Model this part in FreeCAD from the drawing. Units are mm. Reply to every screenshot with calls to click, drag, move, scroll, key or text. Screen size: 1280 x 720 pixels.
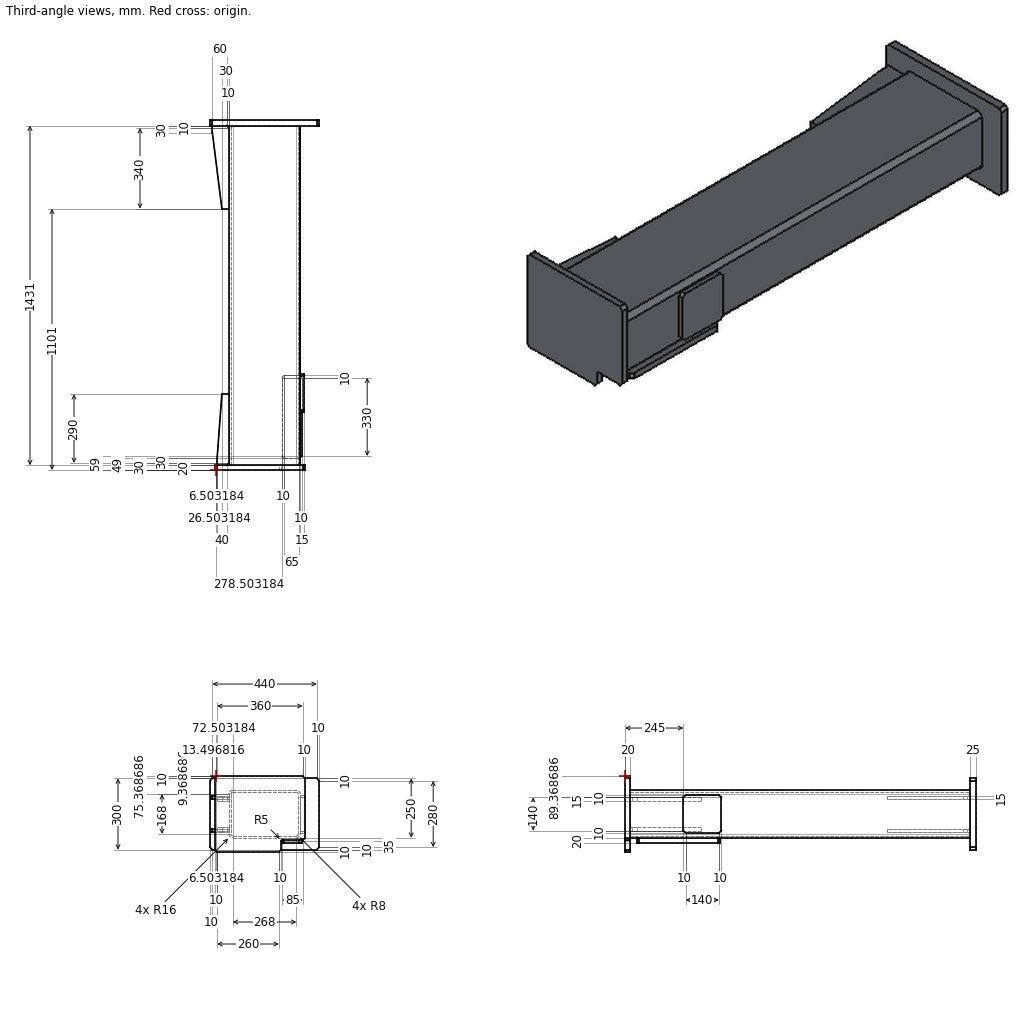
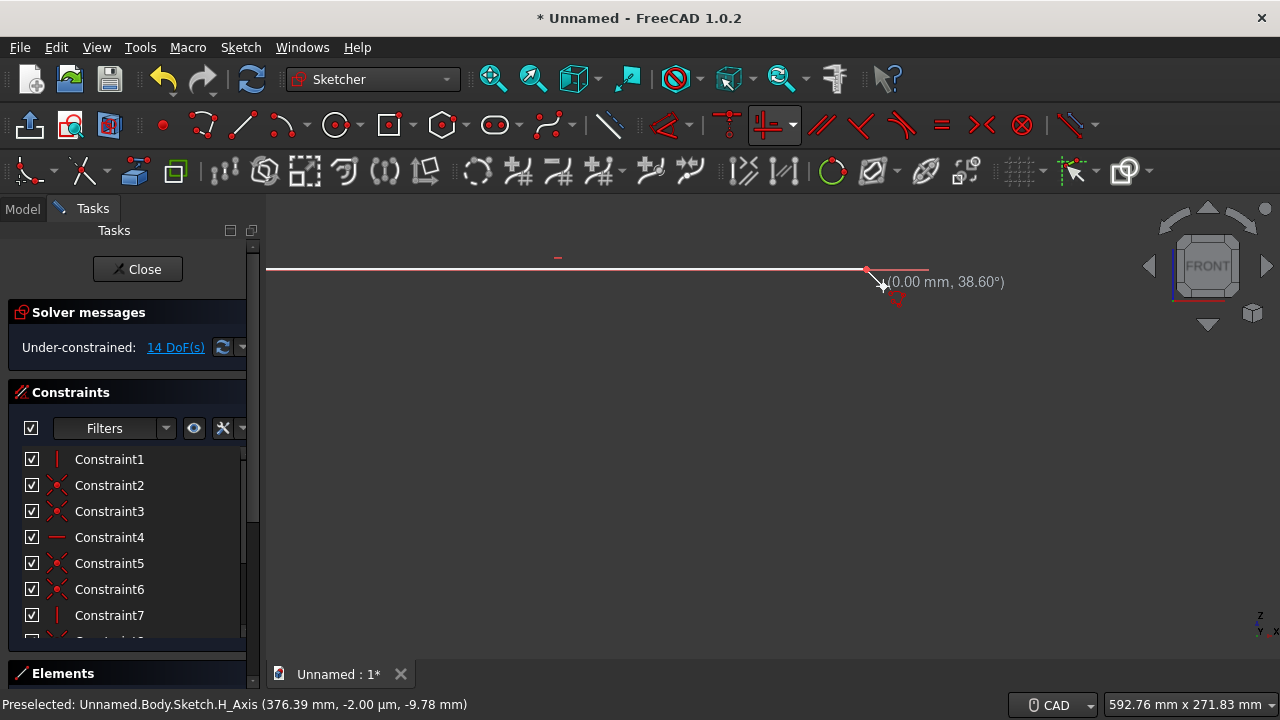
scroll(882, 285, down, 3)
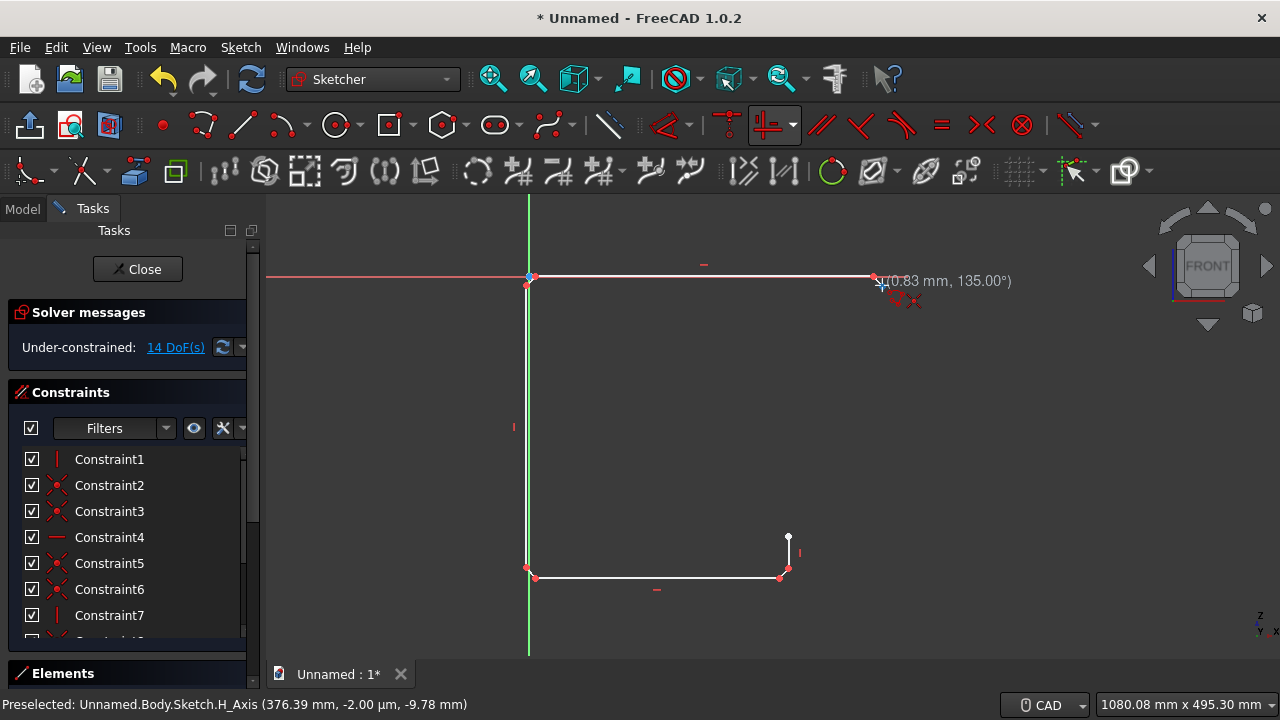
click(883, 520)
click(874, 530)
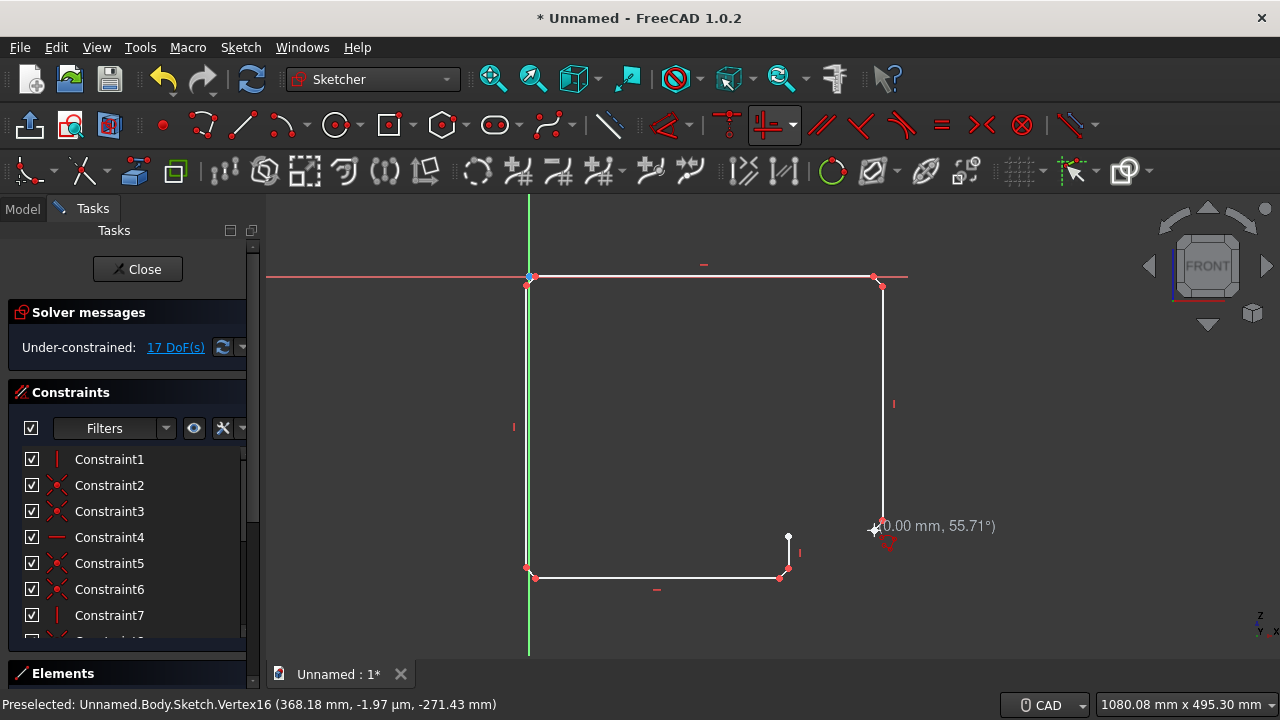
scroll(794, 530, up, 5)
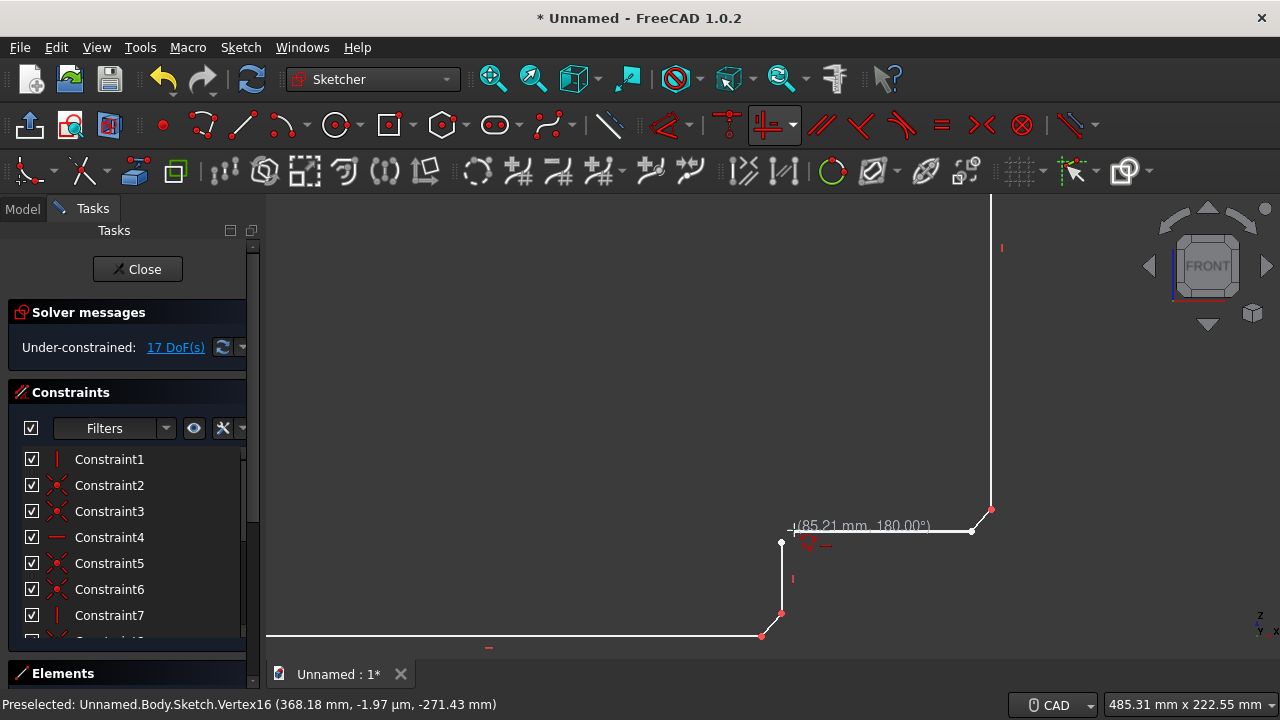
click(792, 529)
right_click(792, 529)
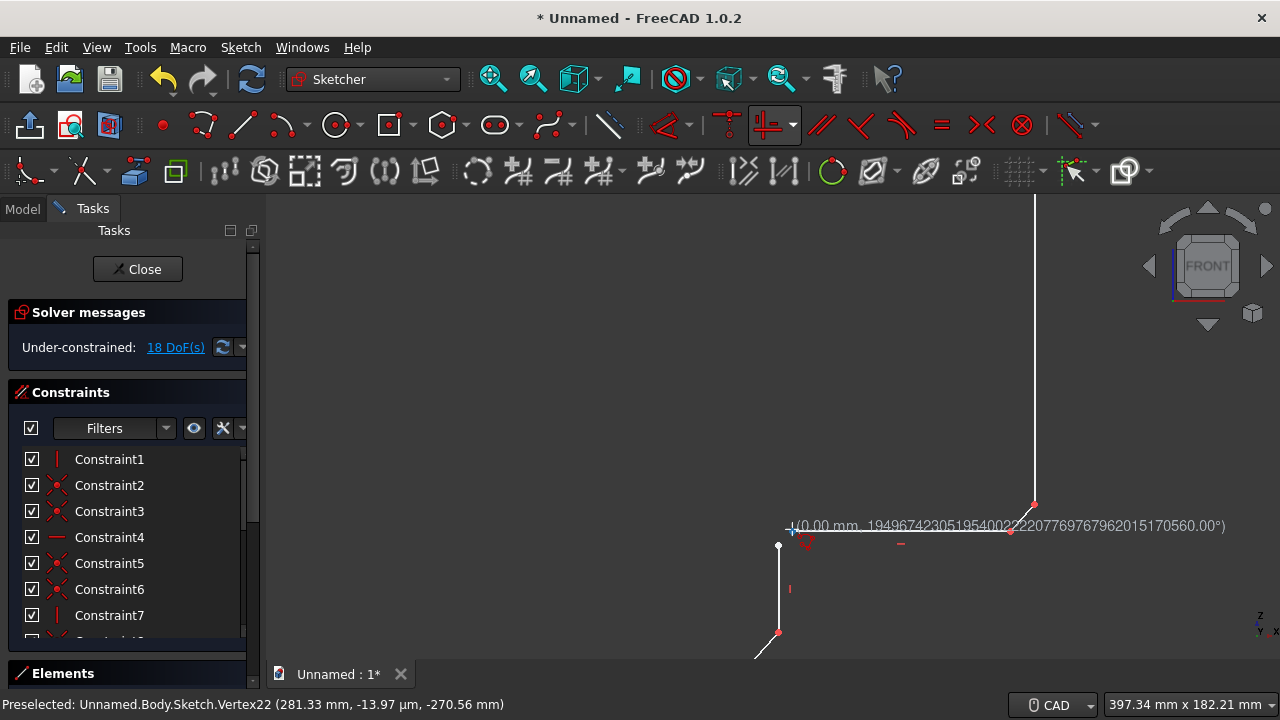
key(g)
key(3)
key(a)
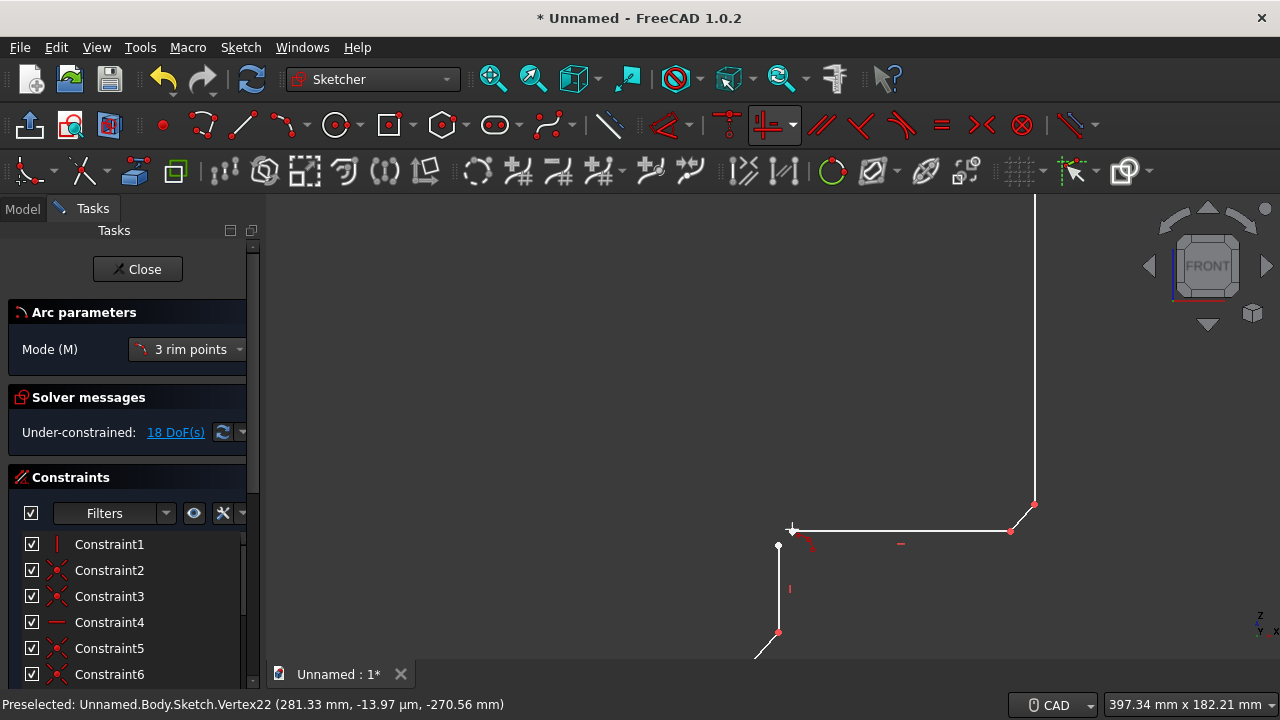
click(792, 531)
click(779, 545)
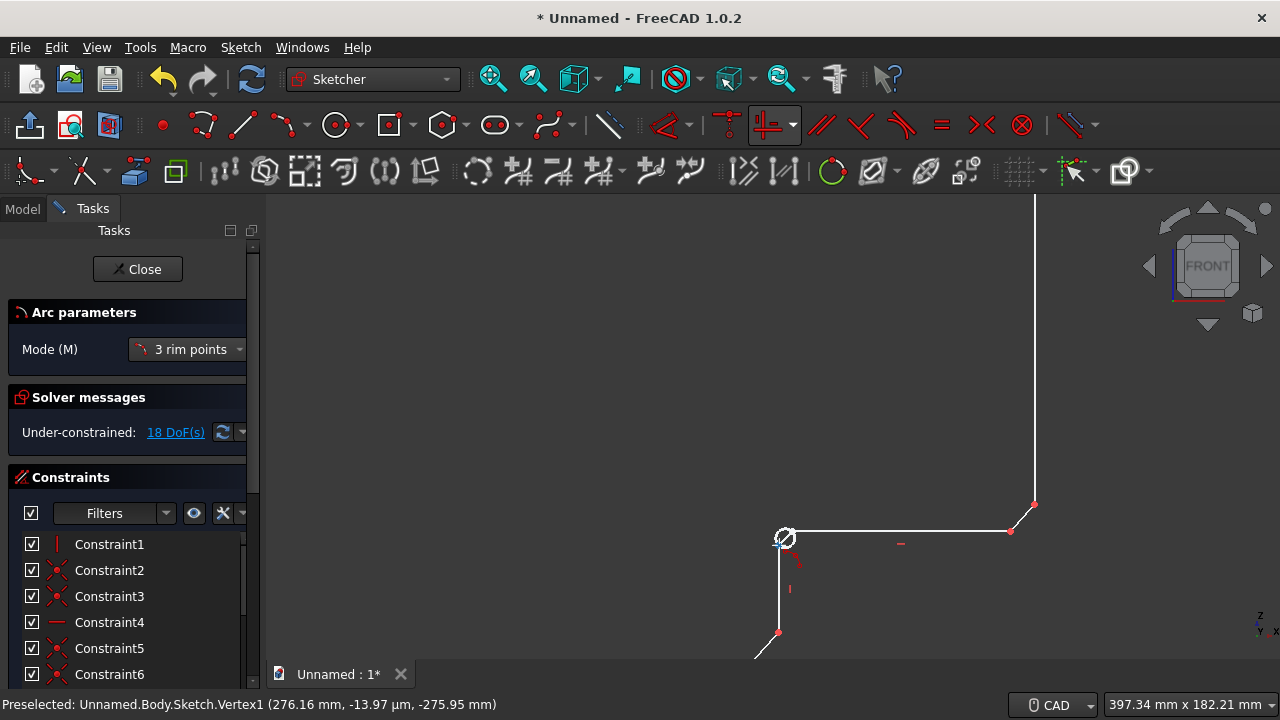
scroll(783, 532, up, 8)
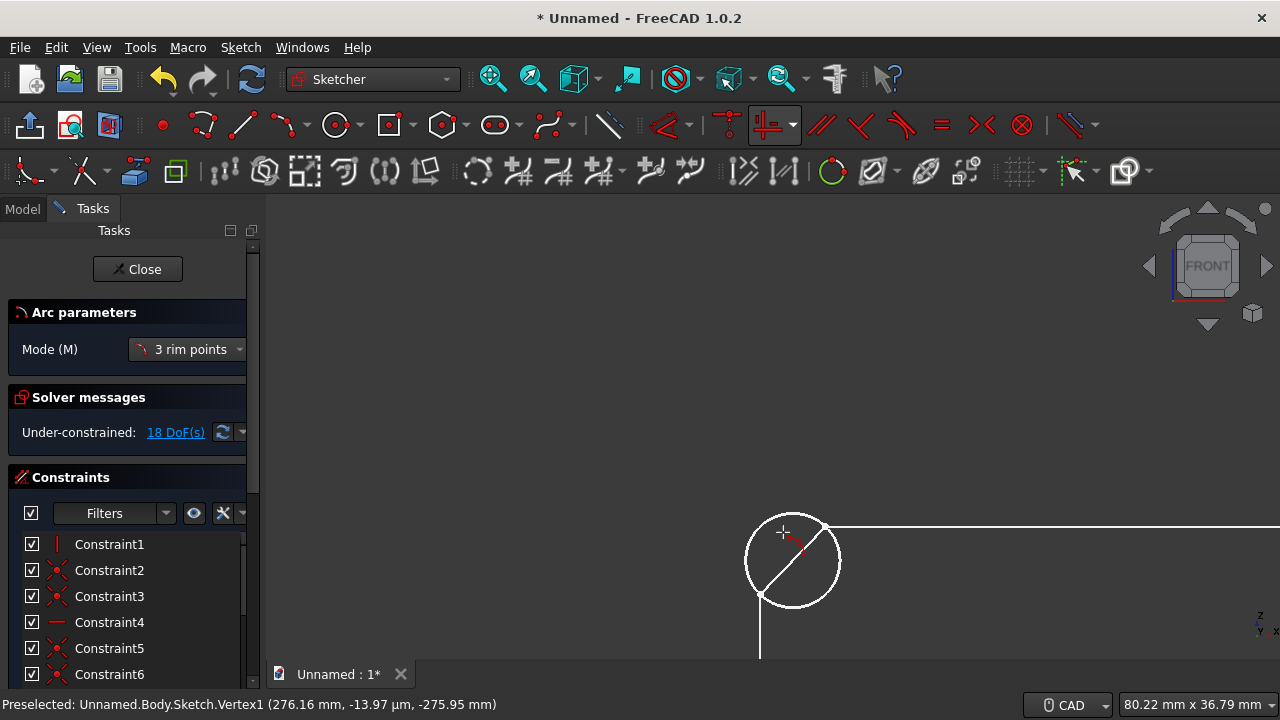
click(783, 530)
key(Escape)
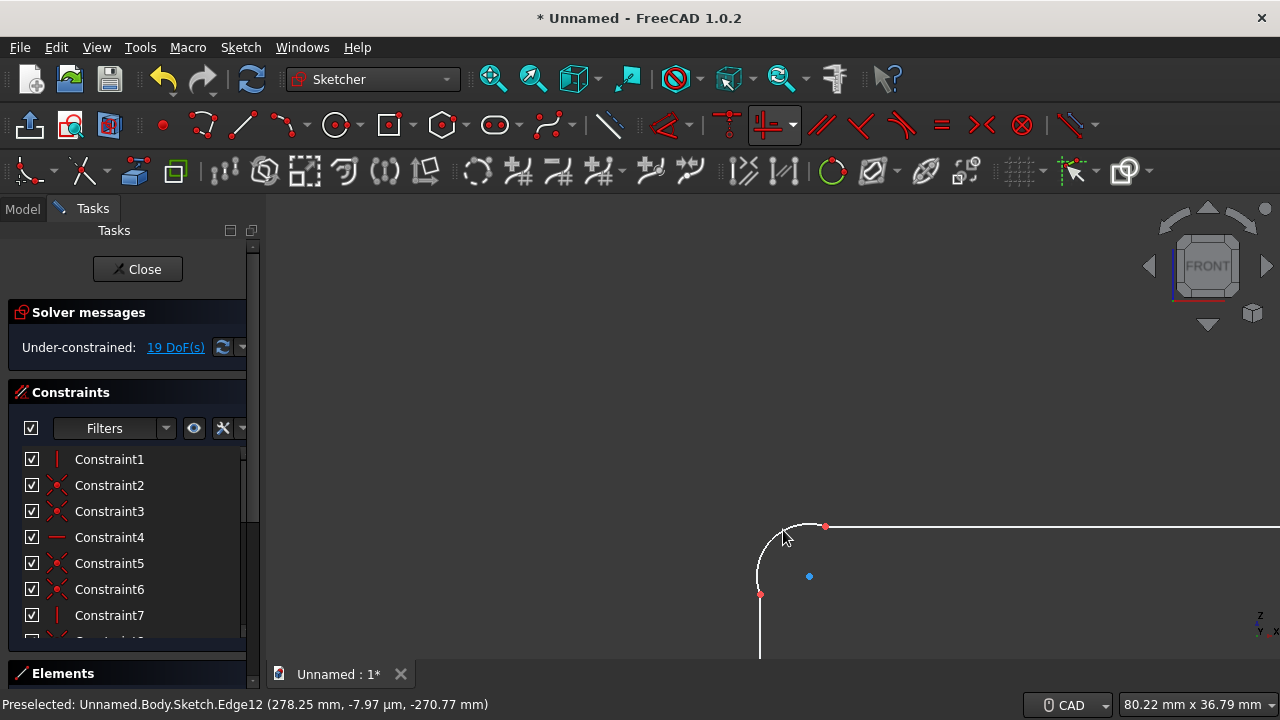
scroll(791, 531, down, 13)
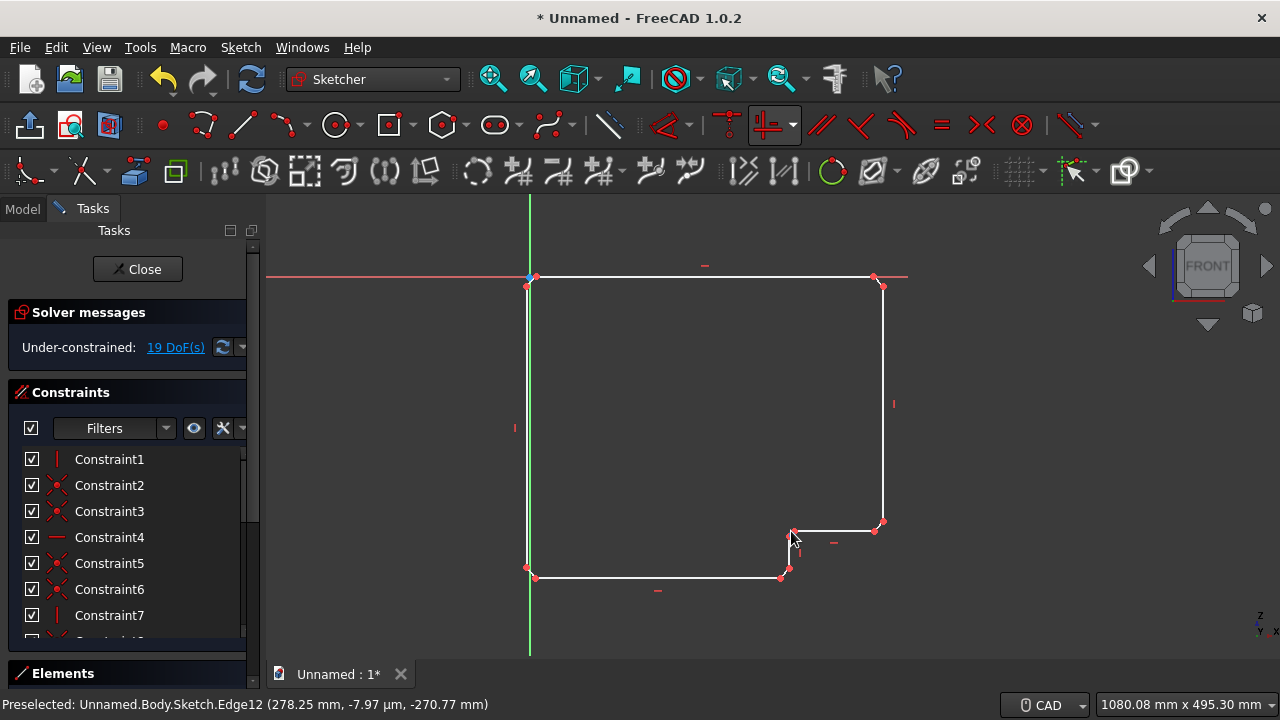
scroll(789, 546, up, 2)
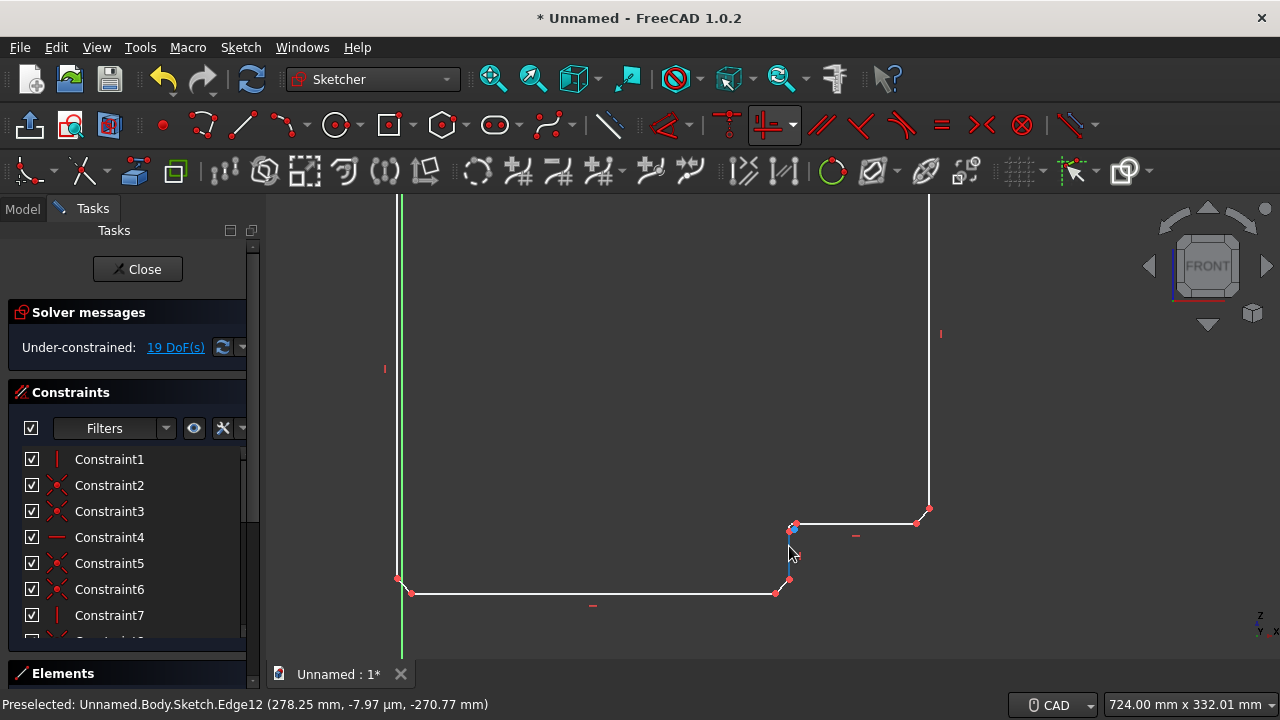
click(789, 546)